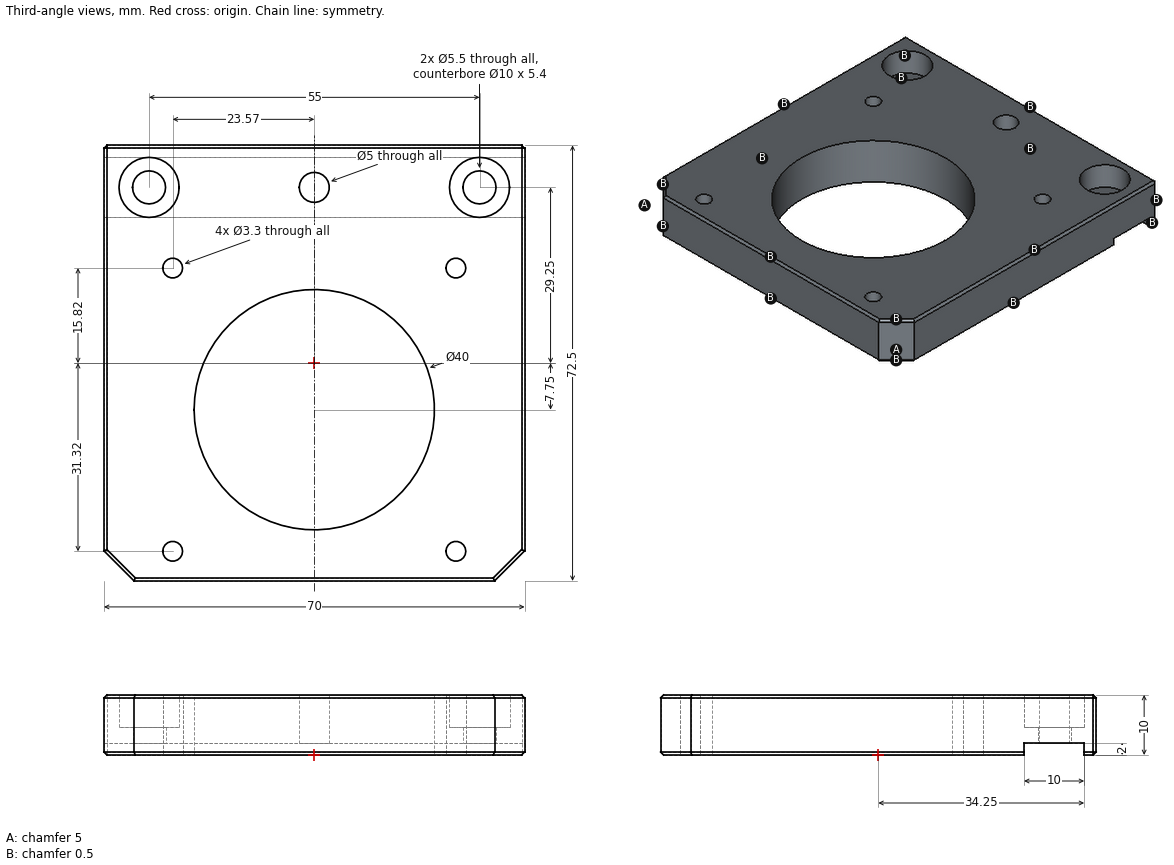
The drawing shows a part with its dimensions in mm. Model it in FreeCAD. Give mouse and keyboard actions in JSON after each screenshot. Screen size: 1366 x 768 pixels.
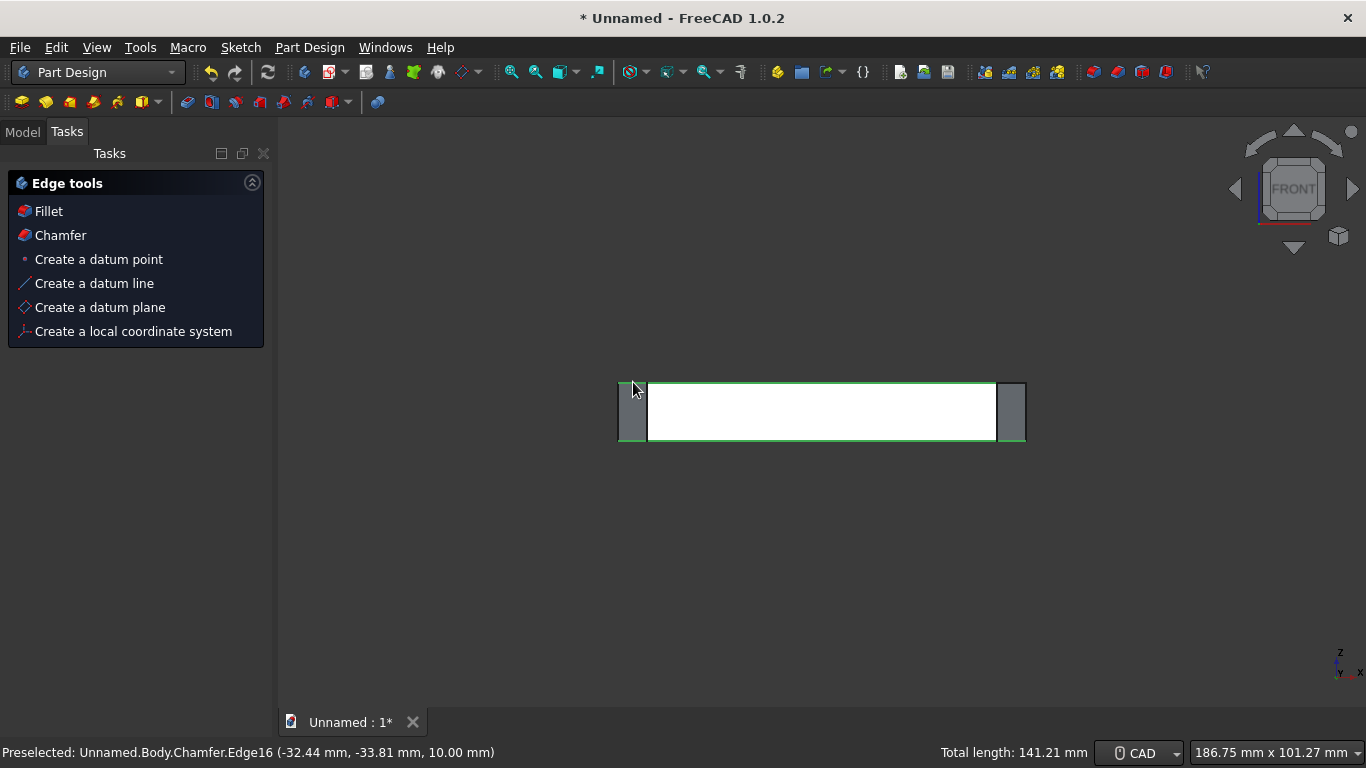
{"action": "left_click", "coordinate": [1011, 382], "text": "ctrl"}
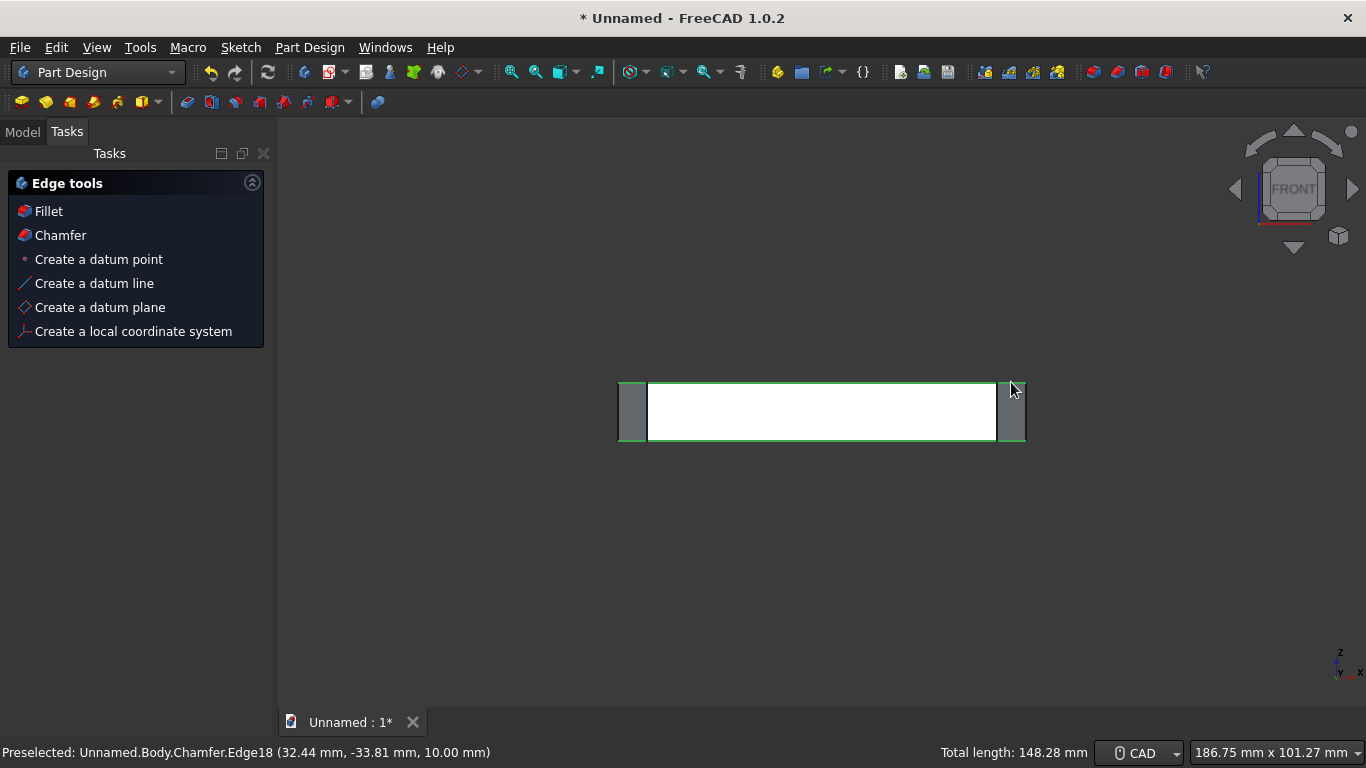
{"action": "key", "text": "0"}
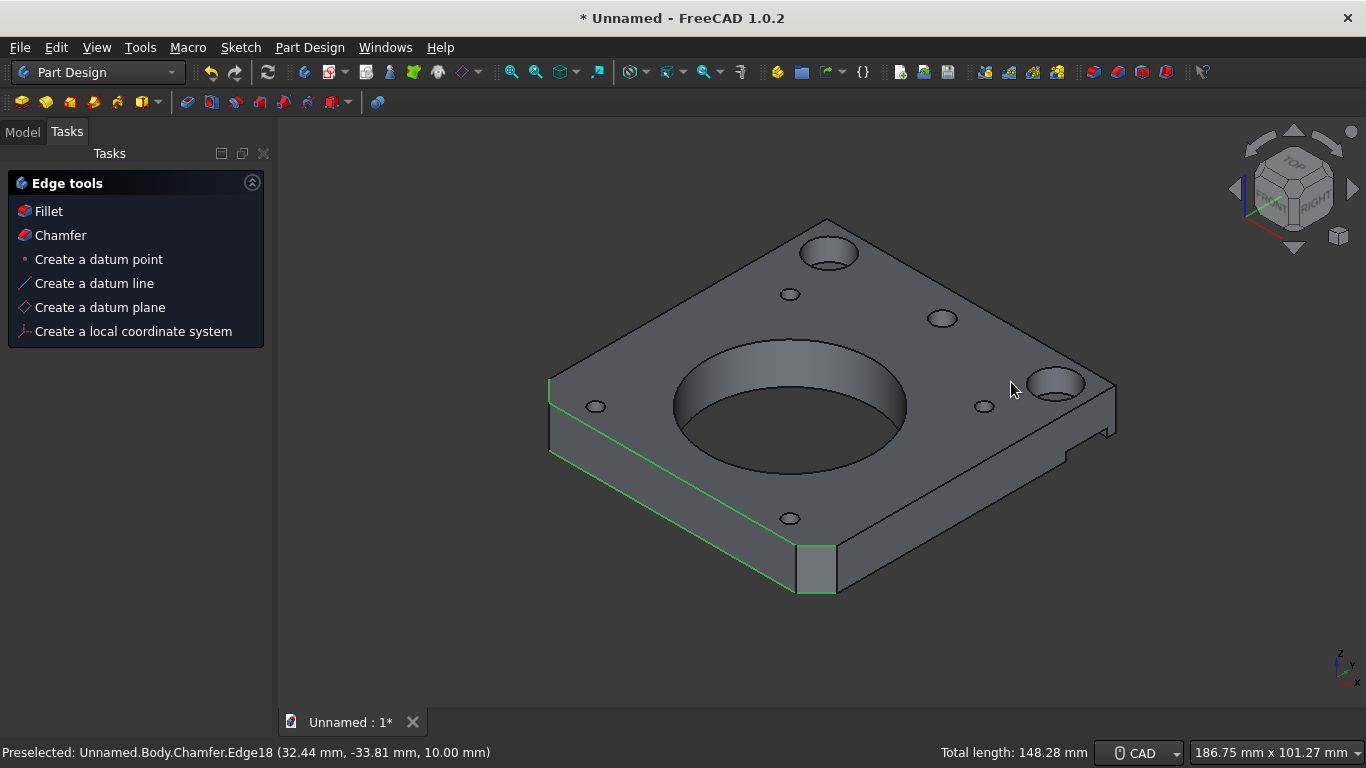
{"action": "left_click", "coordinate": [976, 465], "text": "ctrl"}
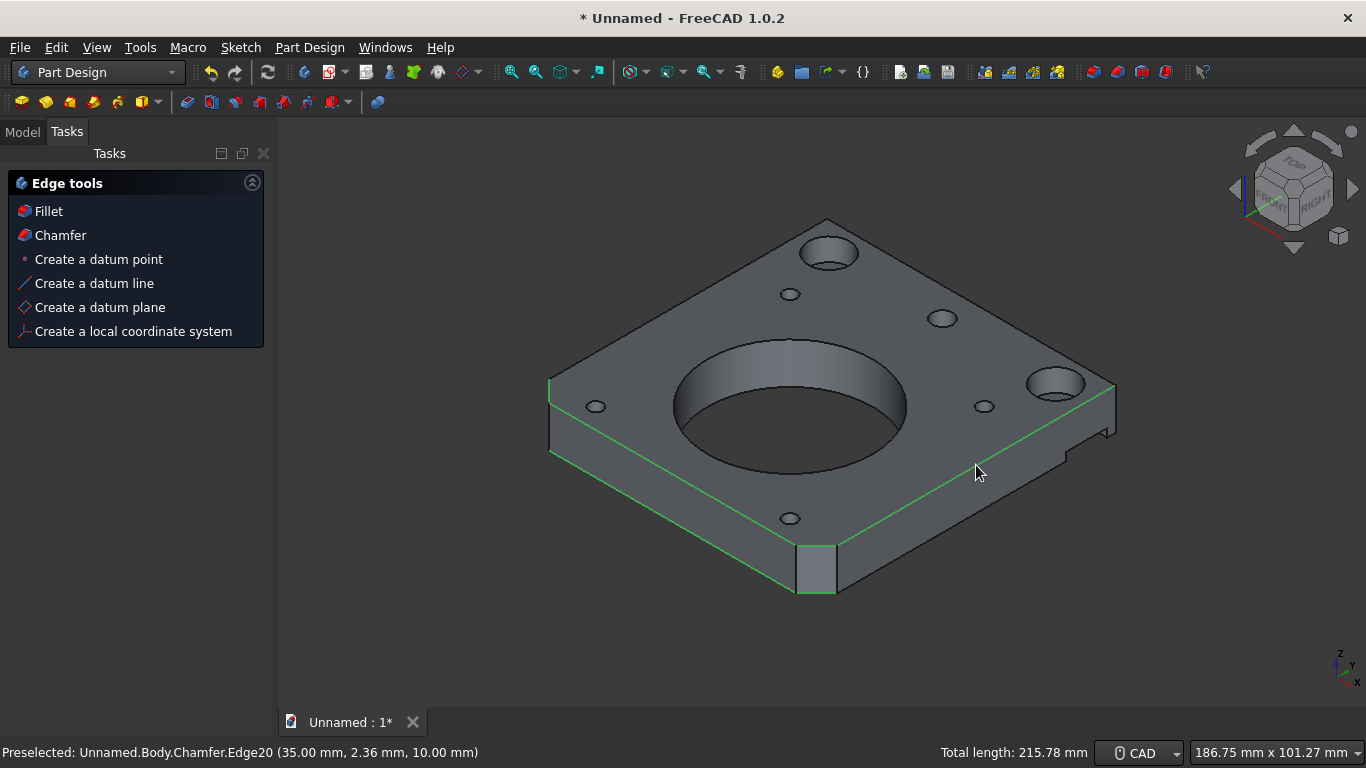
{"action": "key", "text": "2"}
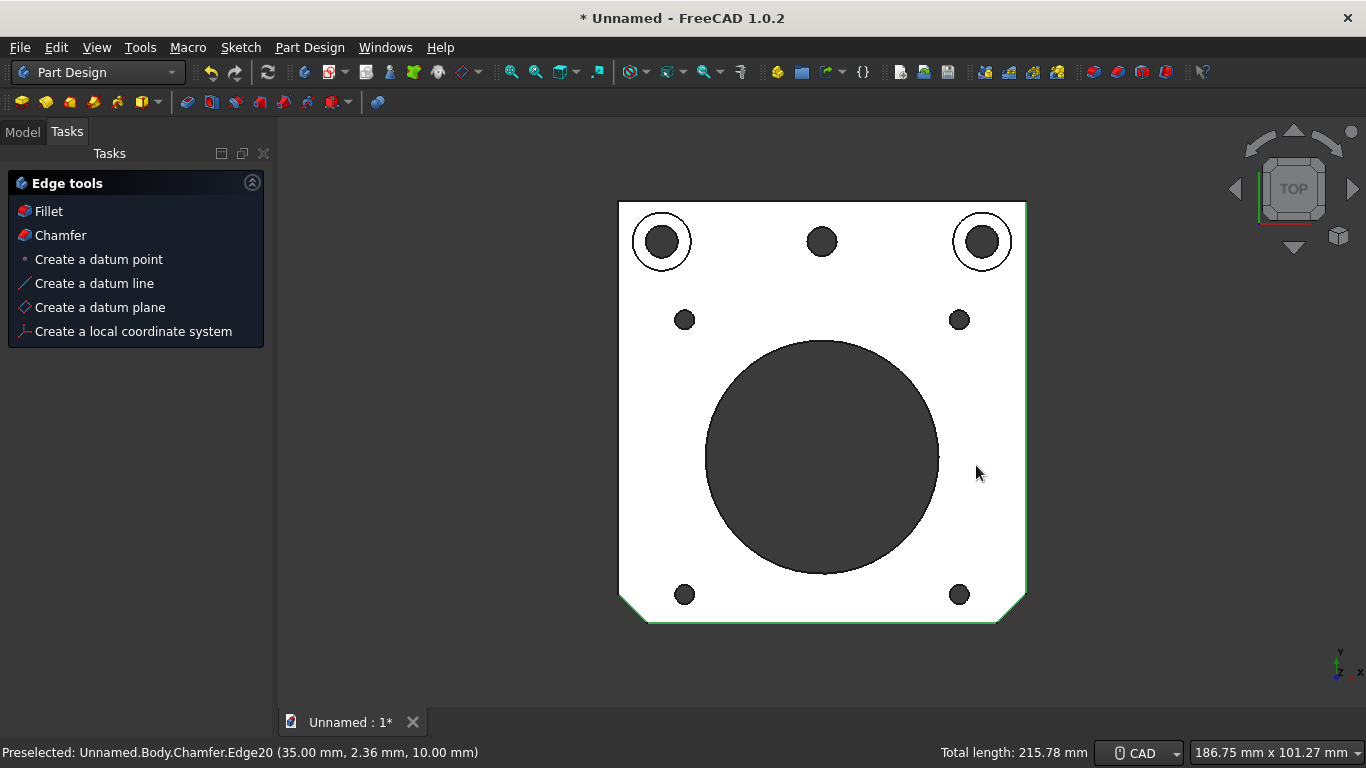
{"action": "left_click", "coordinate": [618, 396], "text": "ctrl"}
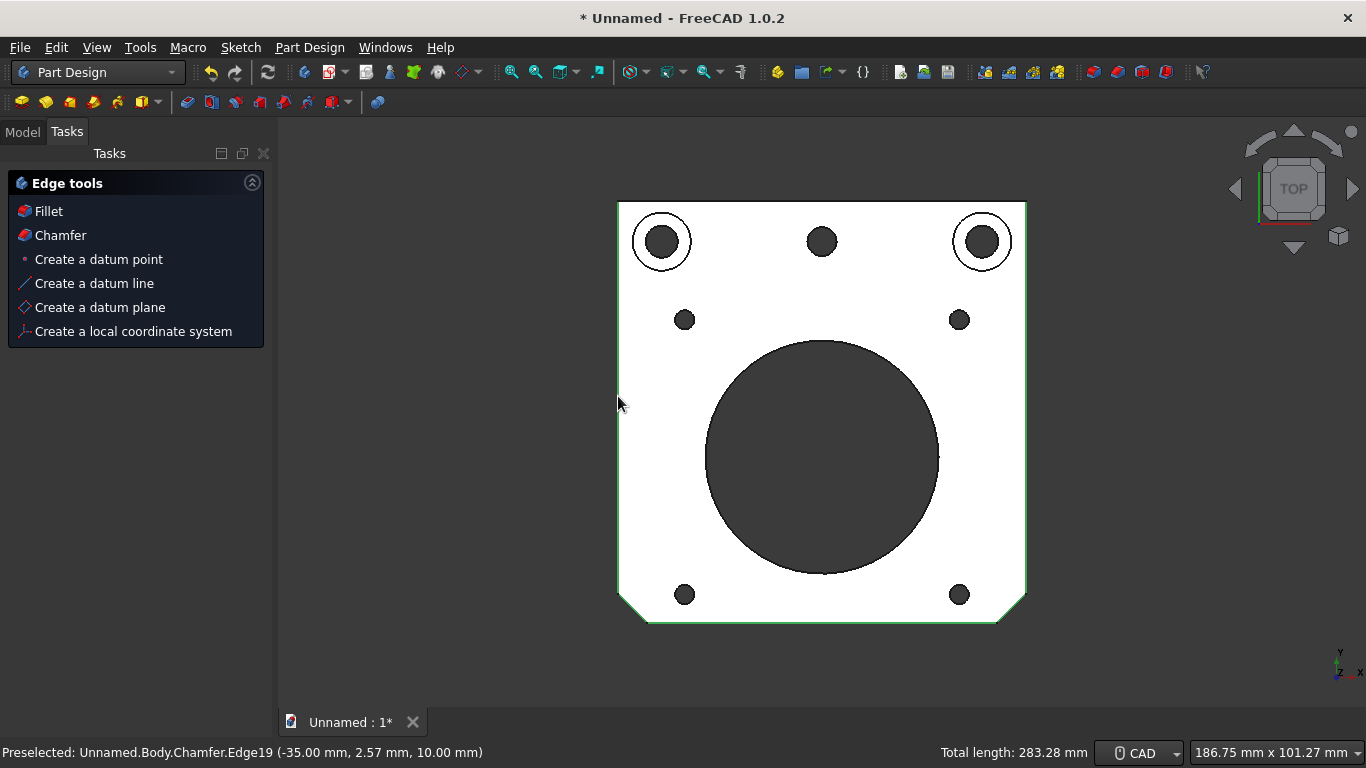
{"action": "key", "text": "1"}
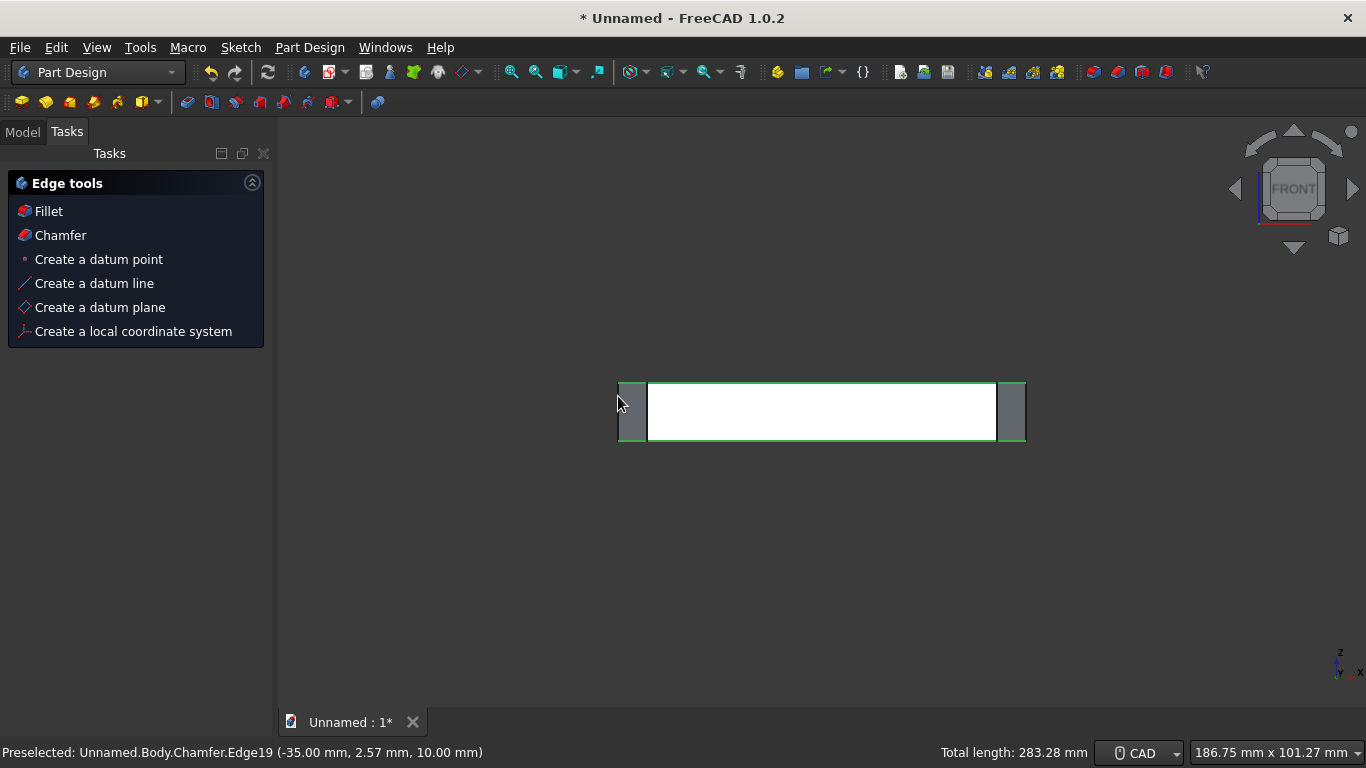
{"action": "key", "text": "v f"}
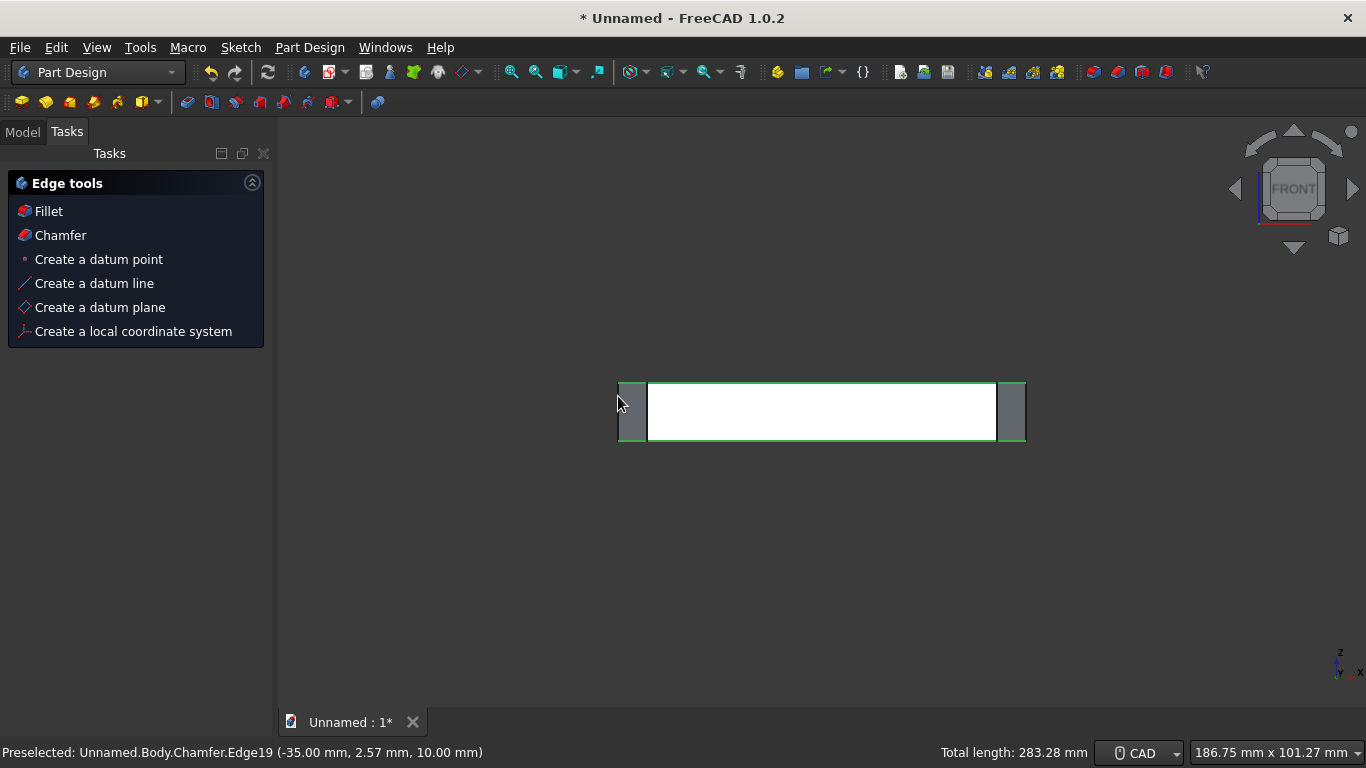
{"action": "key", "text": "3"}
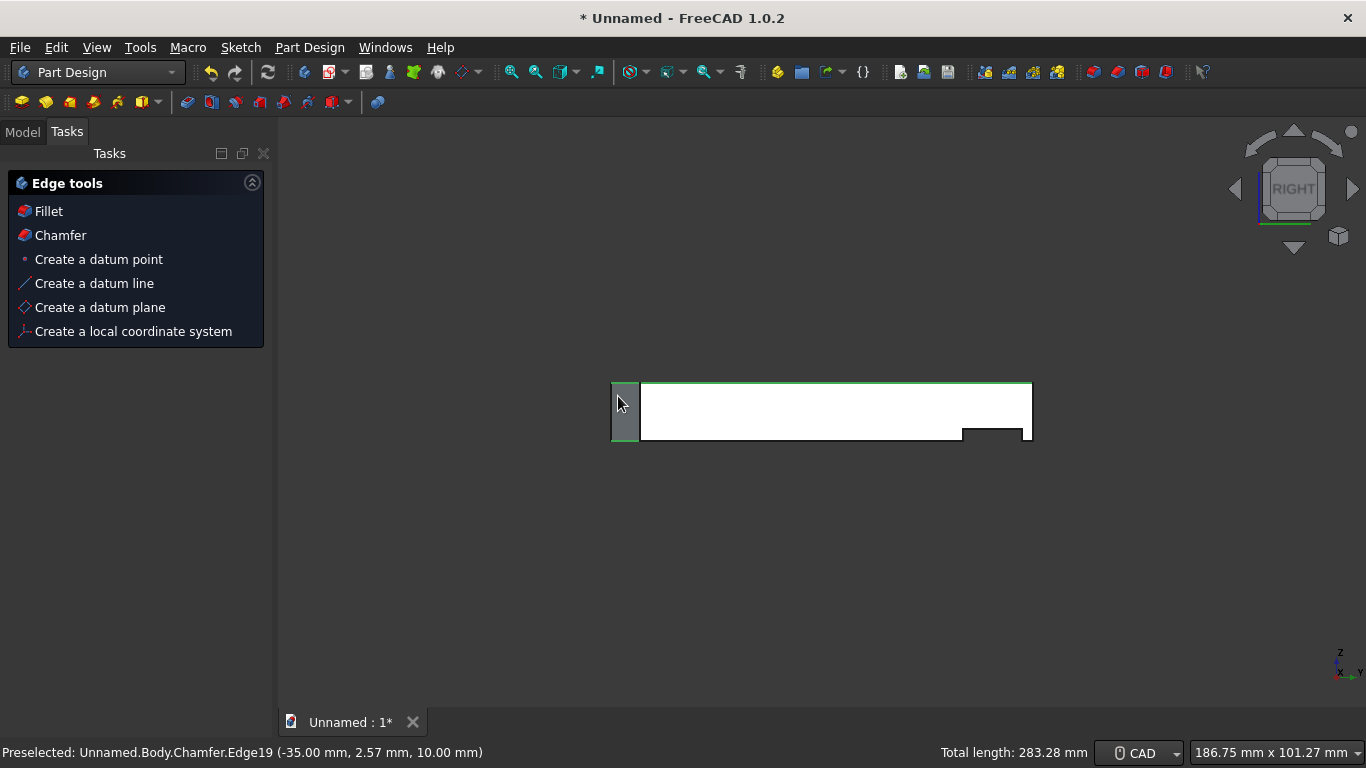
{"action": "left_click", "coordinate": [512, 72]}